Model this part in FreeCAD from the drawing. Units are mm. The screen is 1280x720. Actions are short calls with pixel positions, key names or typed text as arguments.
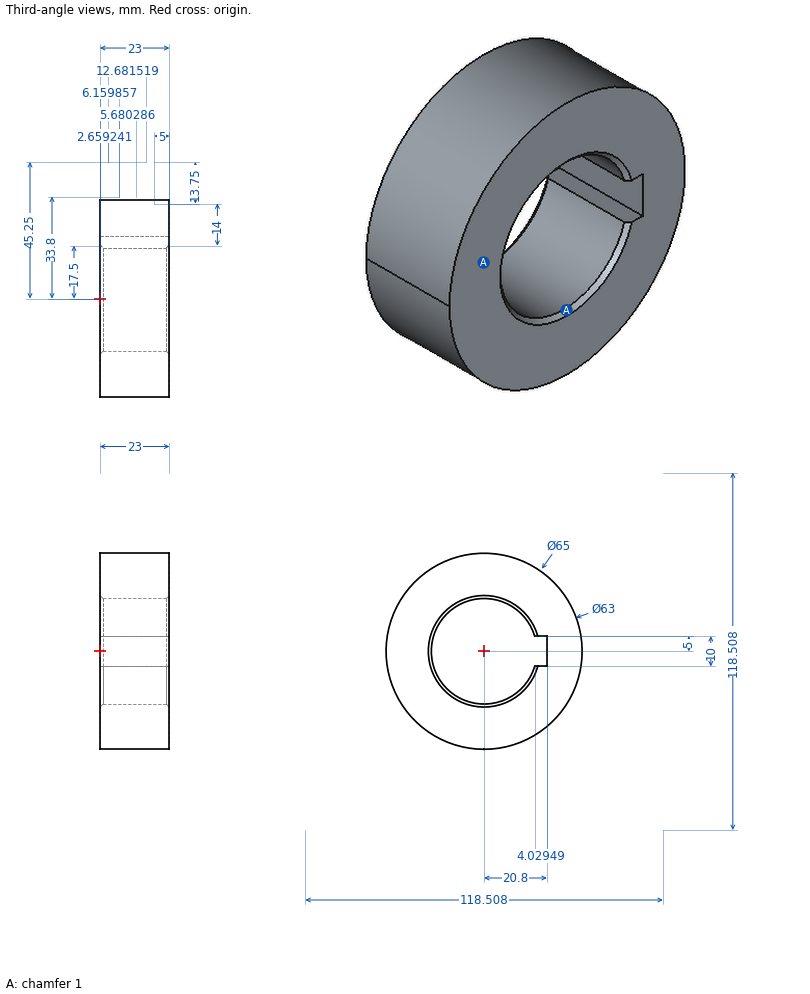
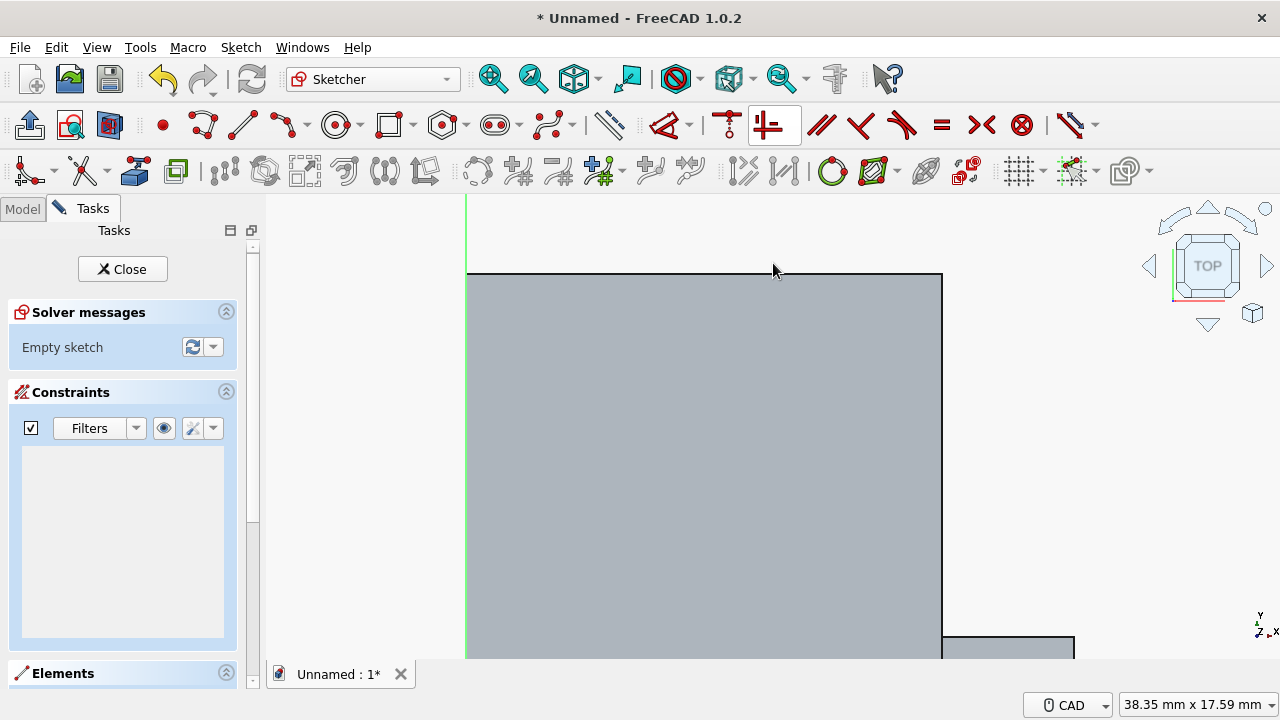
key(g)
key(m)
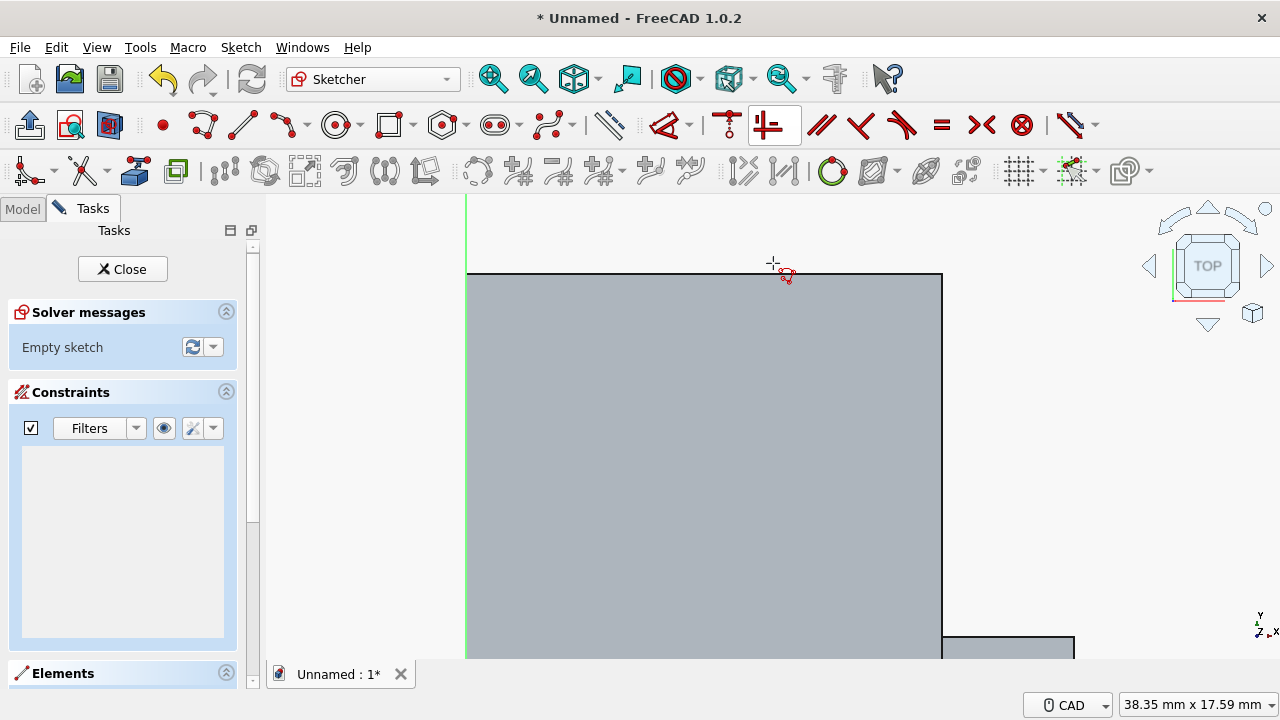
click(629, 576)
click(779, 576)
click(871, 274)
click(536, 274)
click(629, 577)
key(Escape)
key(Escape)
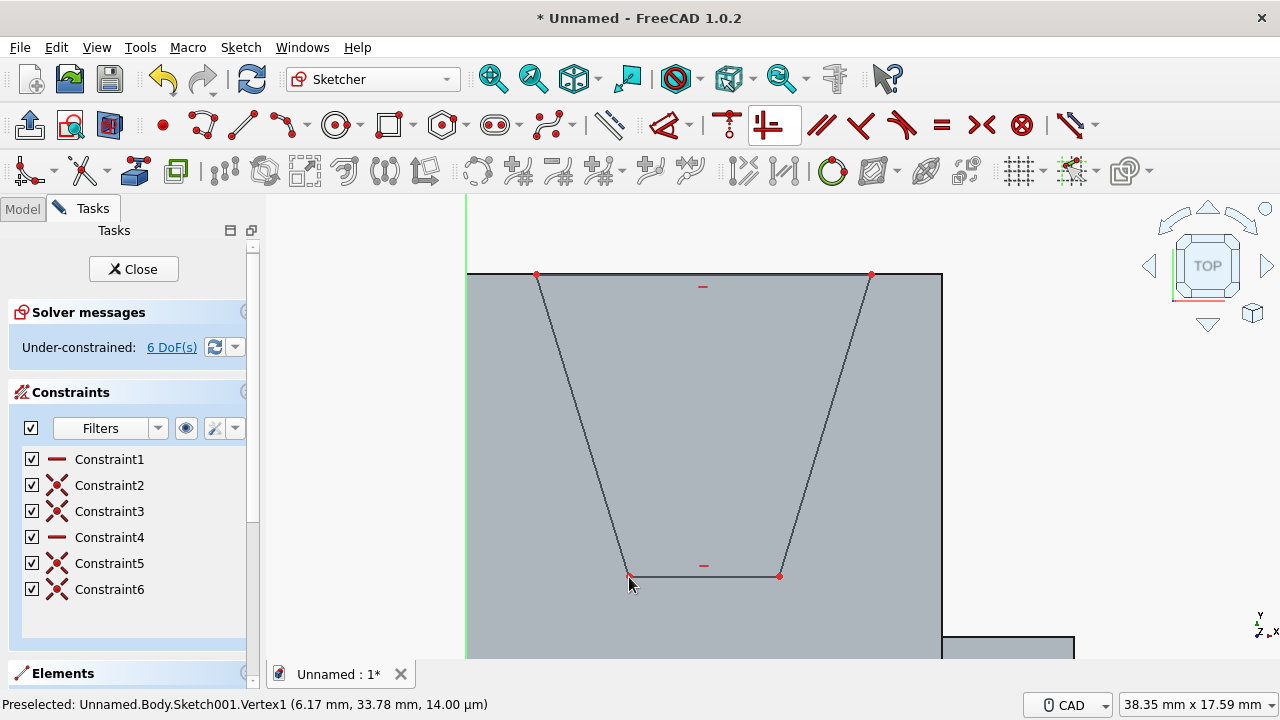
click(664, 126)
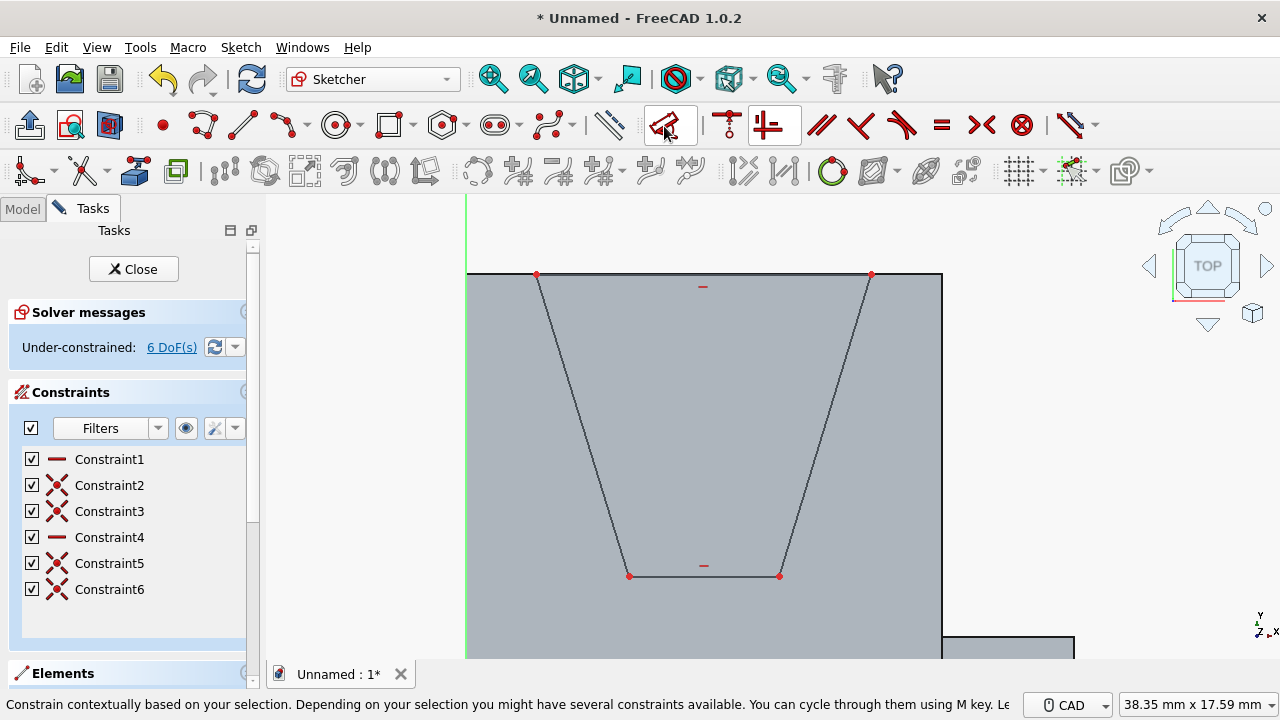
click(629, 577)
click(432, 604)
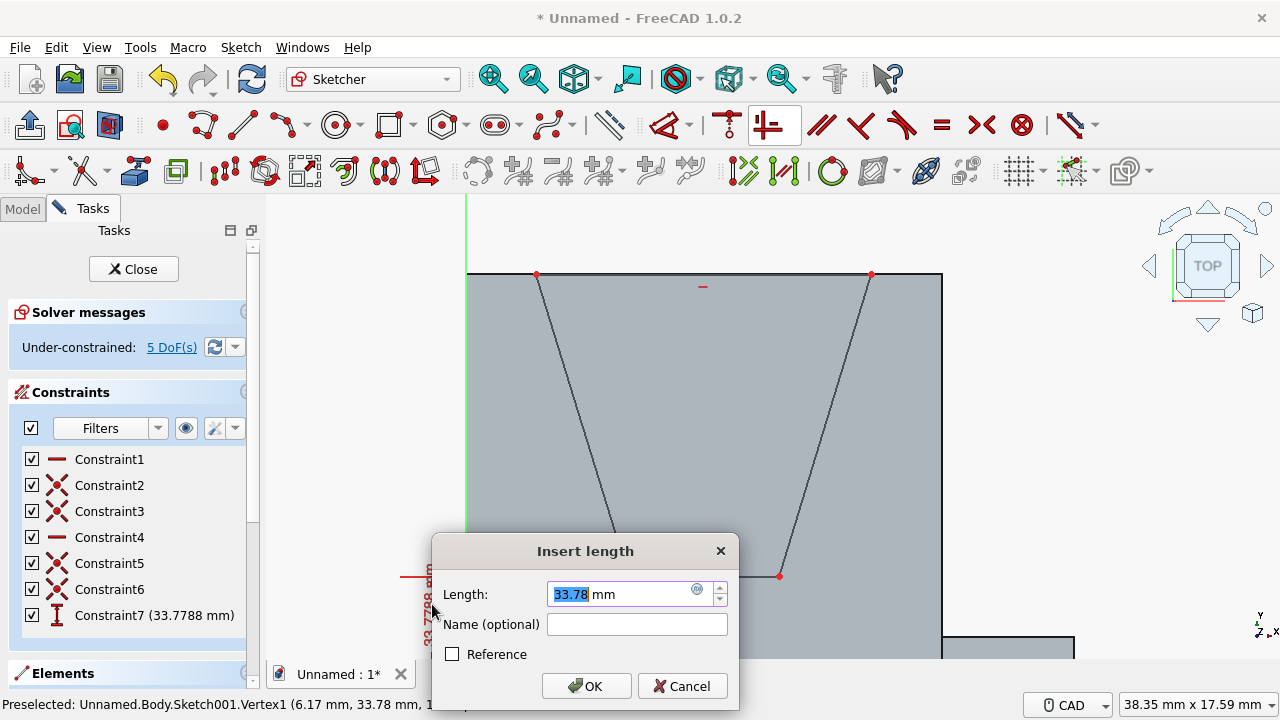
text(33.8)
key(Return)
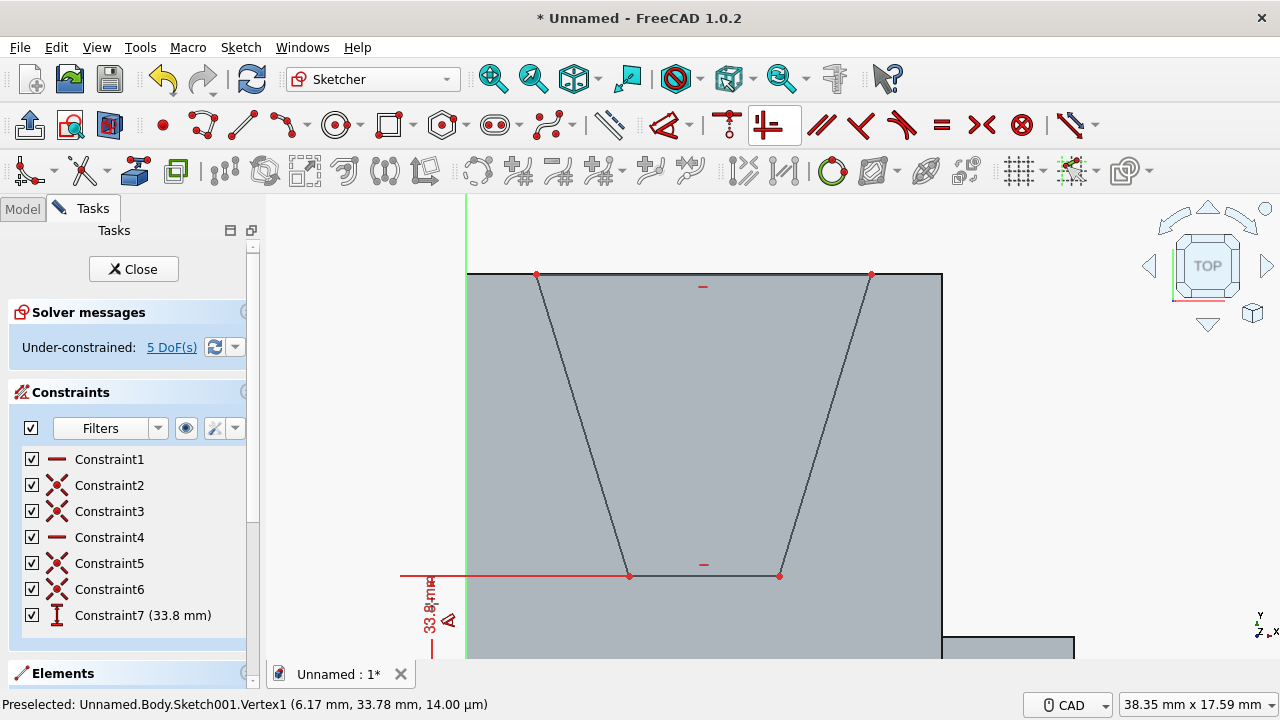
click(871, 275)
click(432, 453)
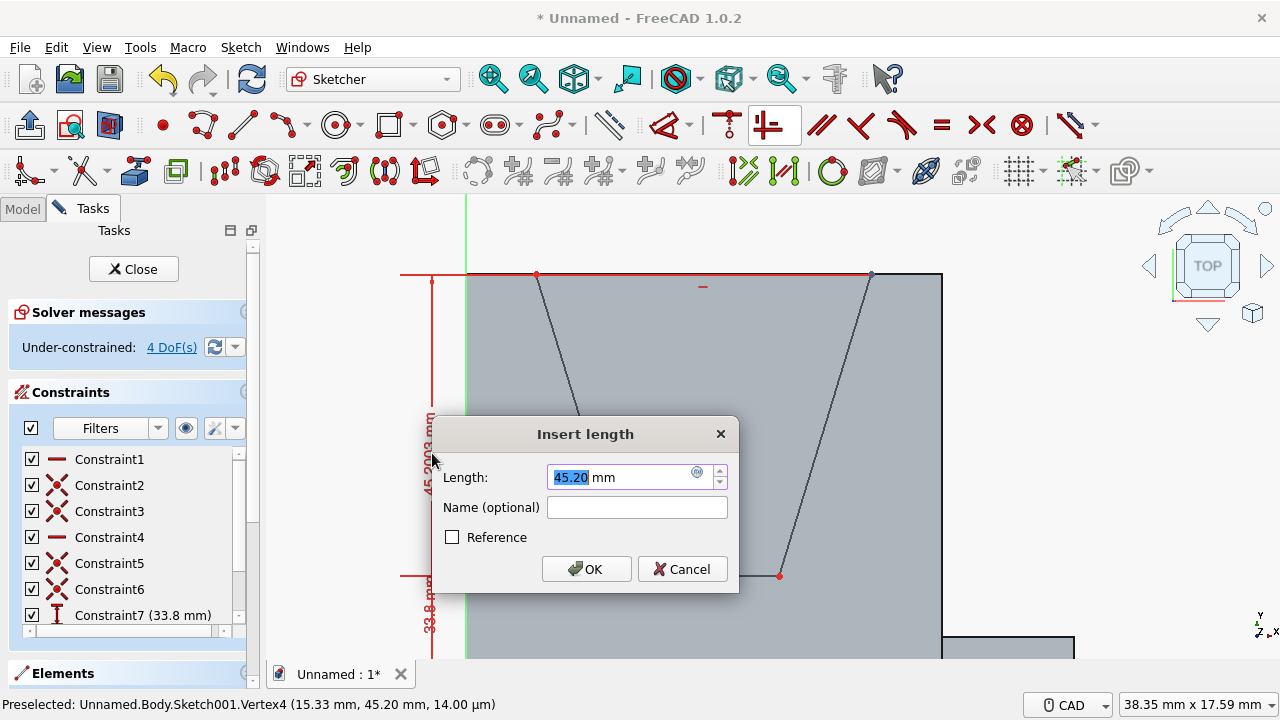
text(45.25)
key(Return)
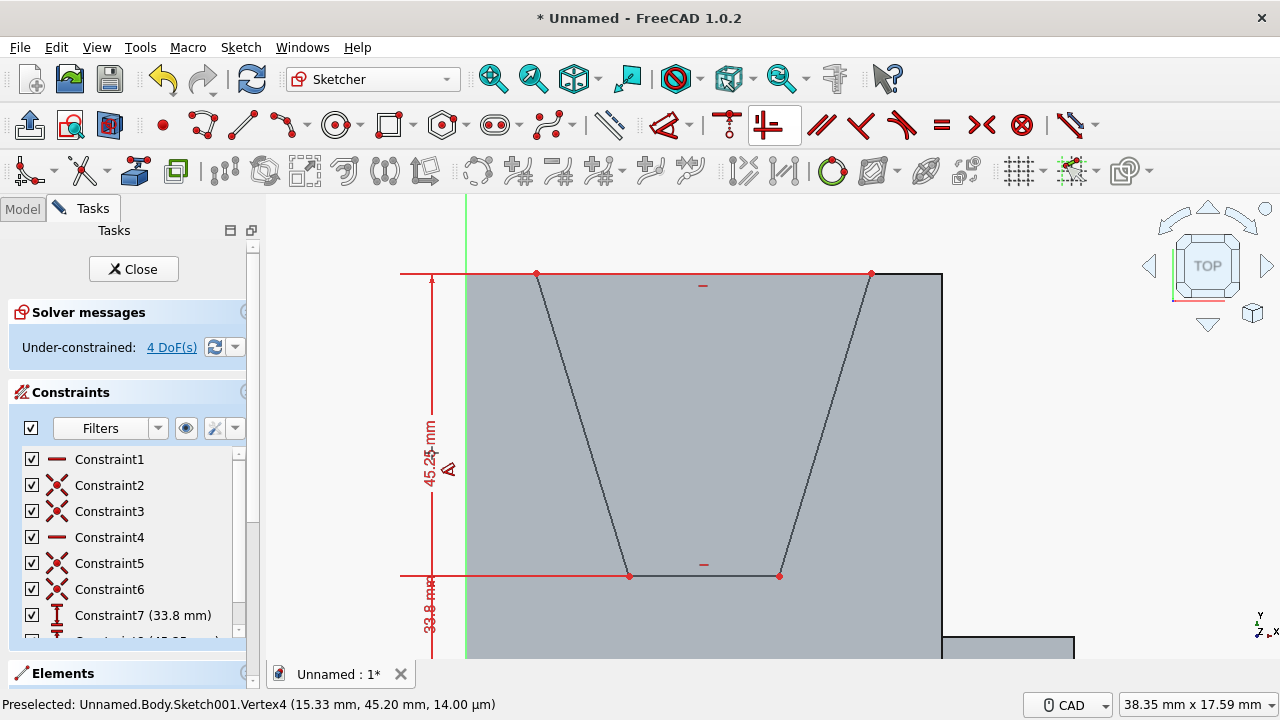
click(674, 576)
click(704, 610)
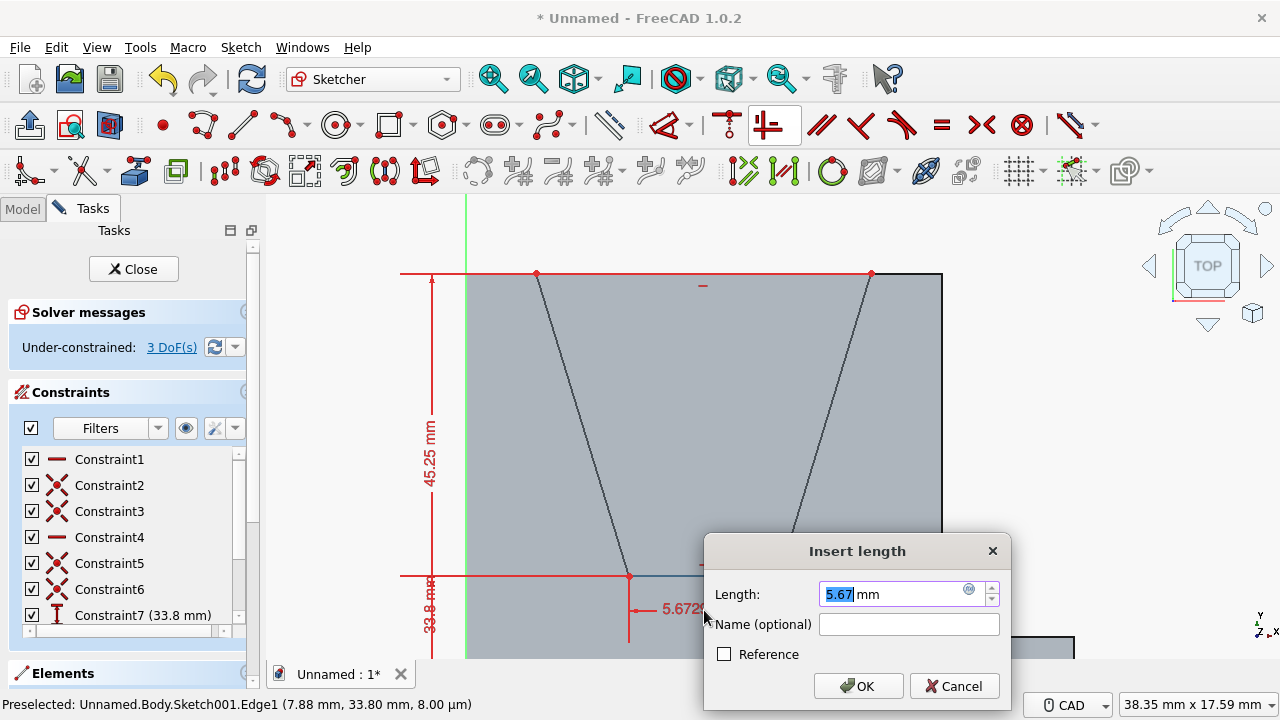
text(5.680286)
key(Return)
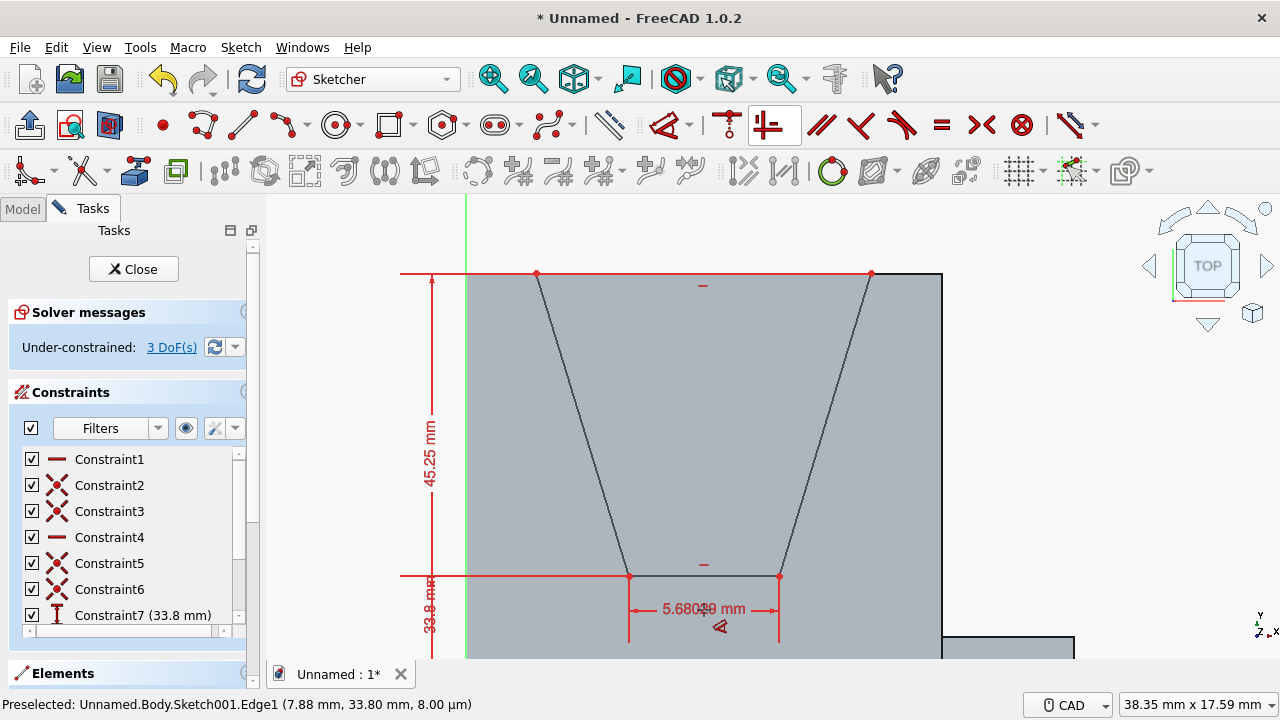
click(771, 274)
click(704, 240)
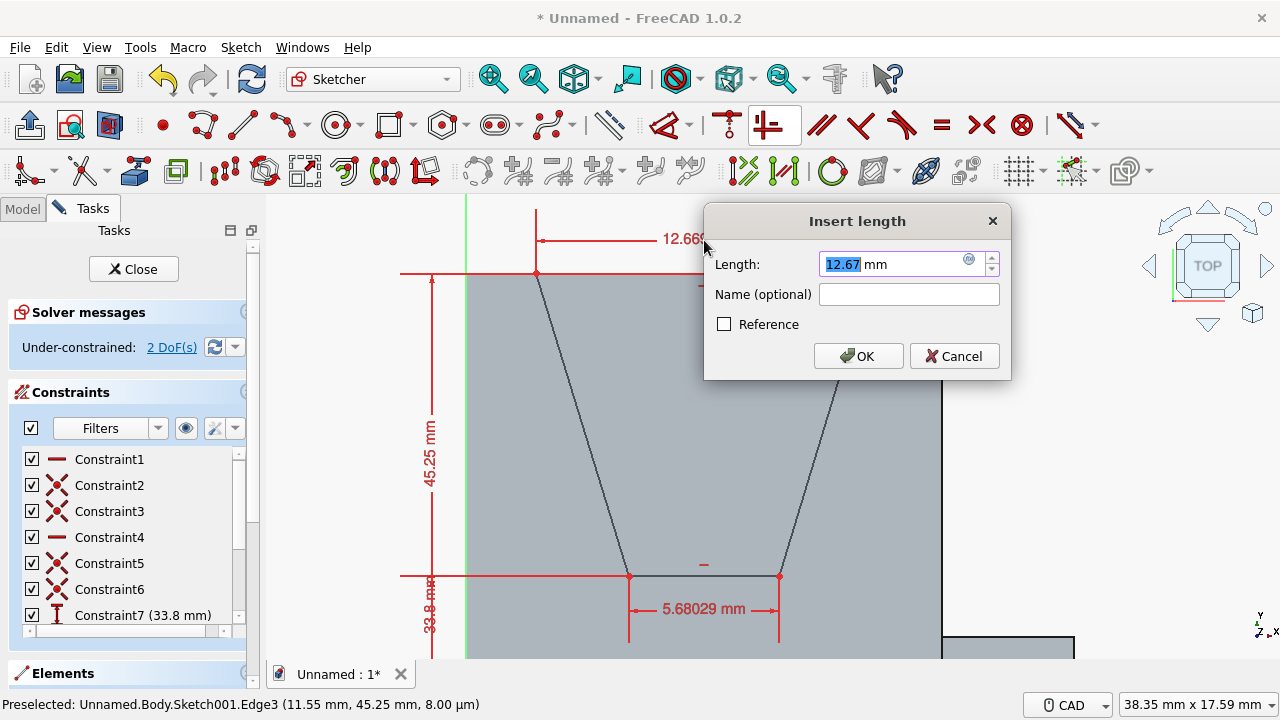
text(12.681519)
key(Return)